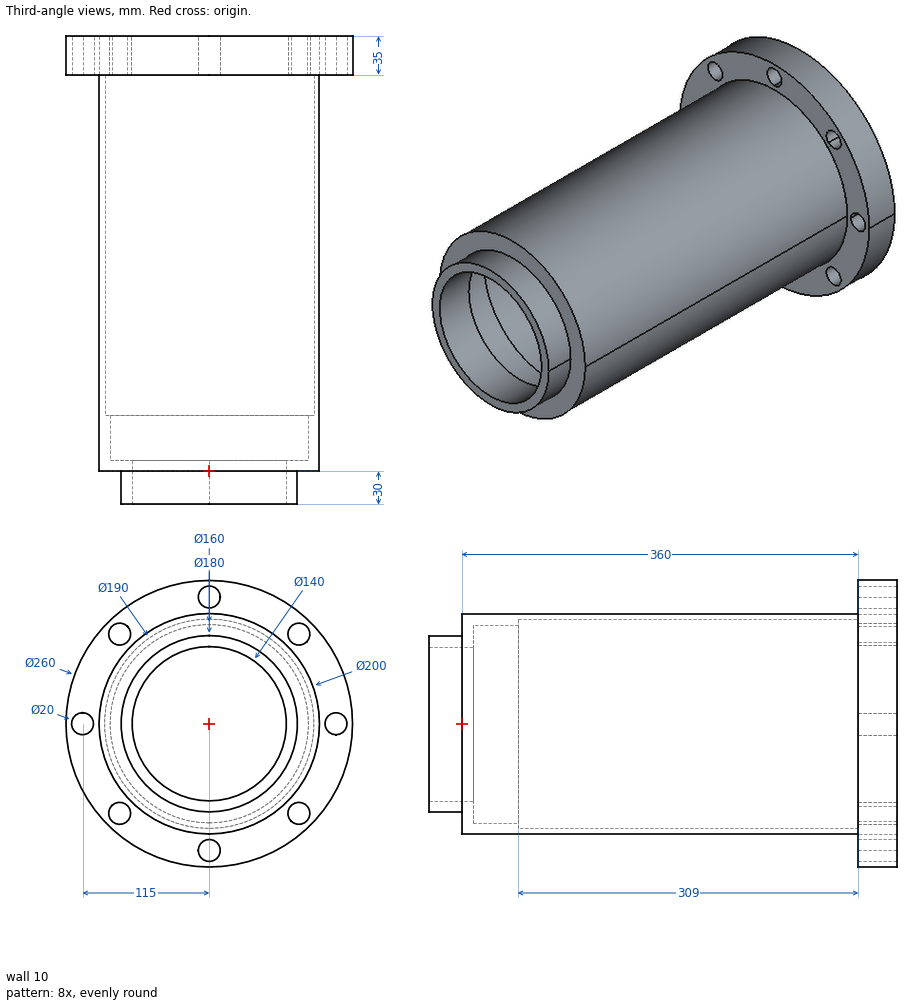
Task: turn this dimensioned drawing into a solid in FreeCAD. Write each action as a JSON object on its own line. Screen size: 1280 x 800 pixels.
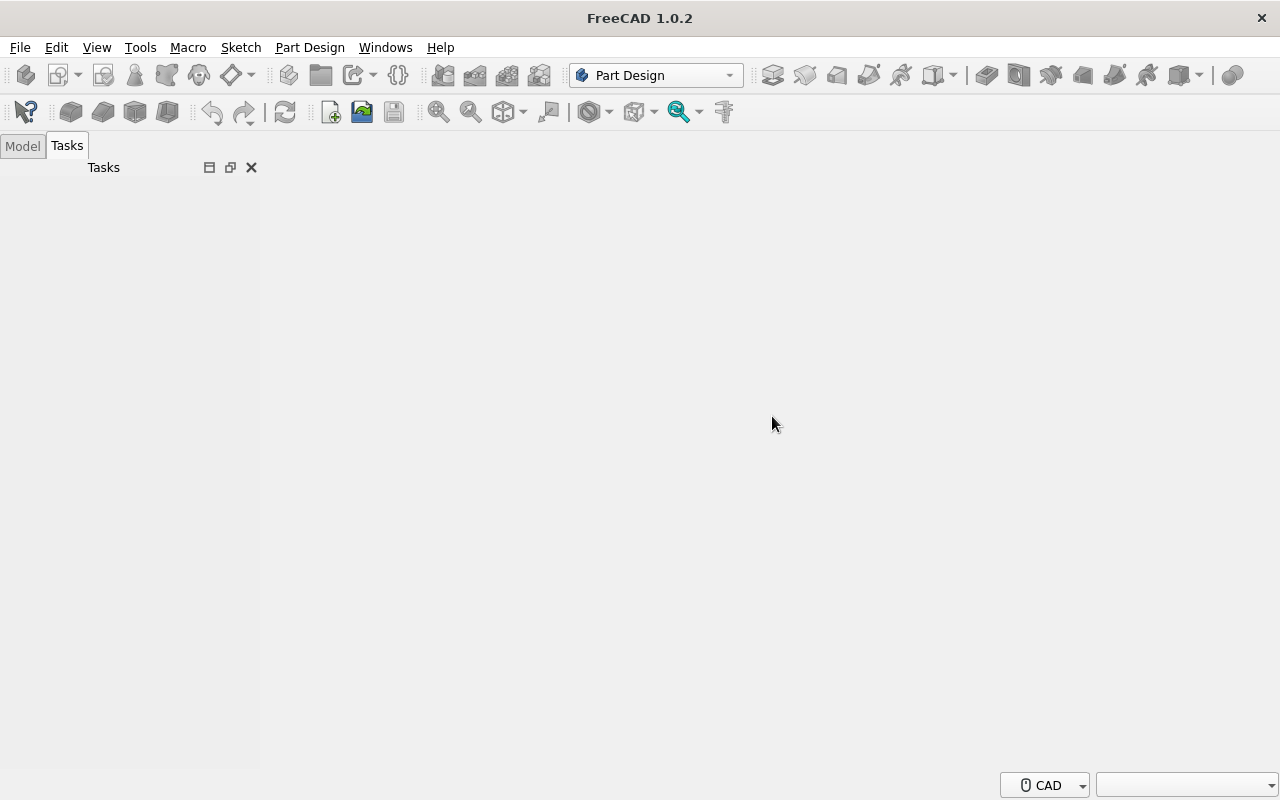
{"action": "key", "text": "ctrl+n"}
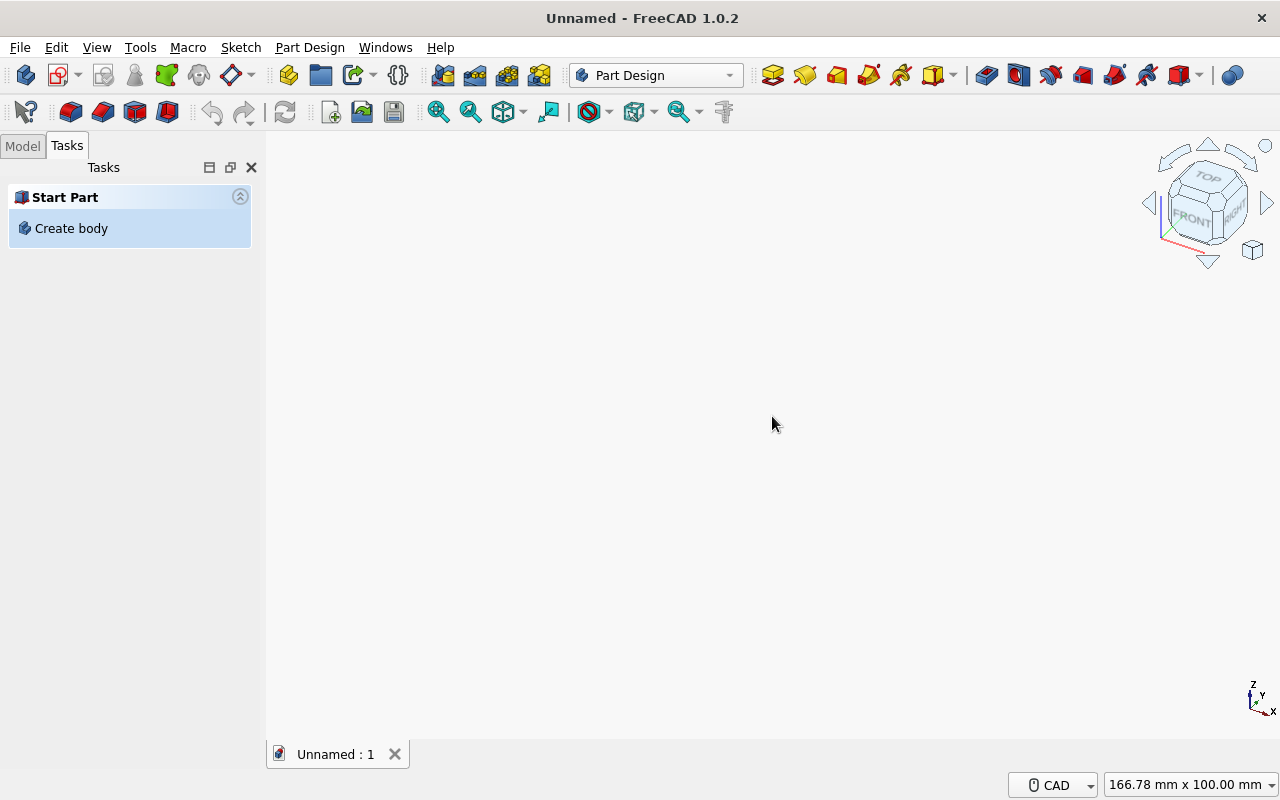
{"action": "left_click", "coordinate": [58, 76]}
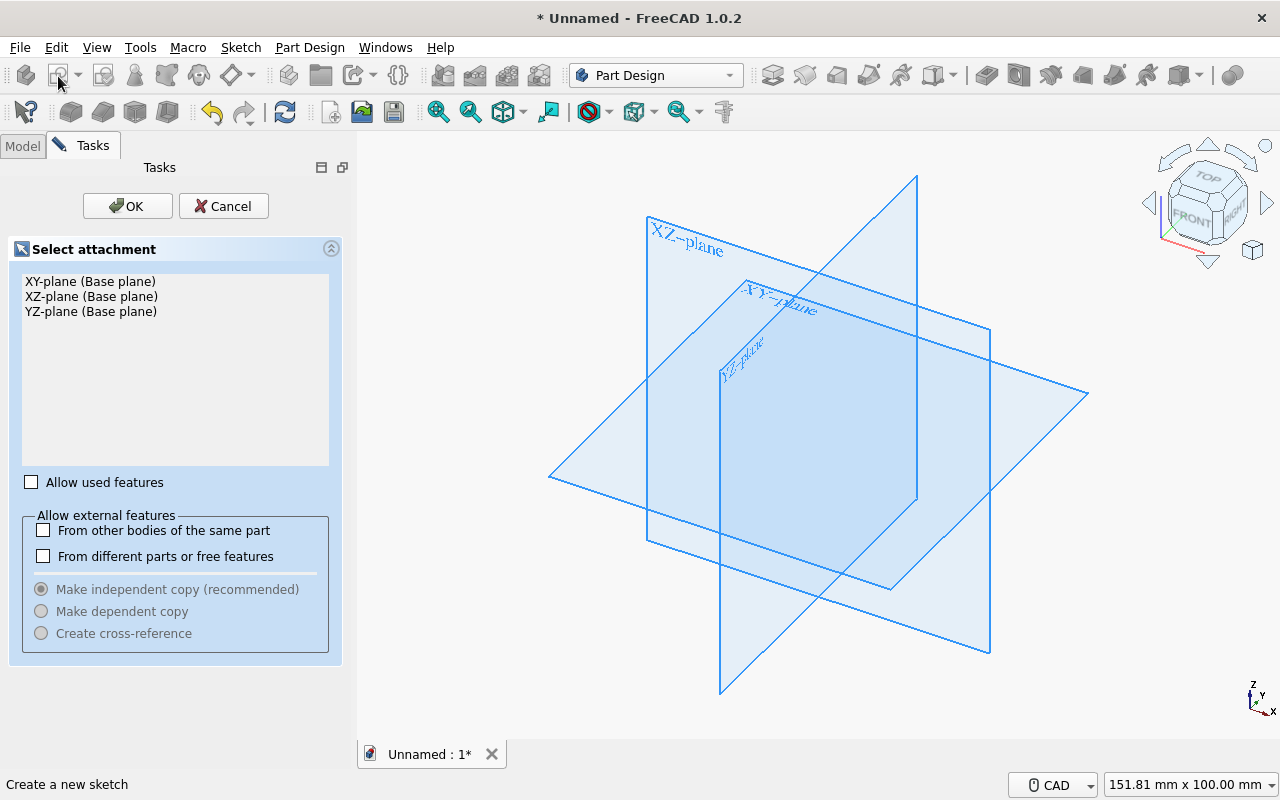
{"action": "left_click", "coordinate": [82, 296]}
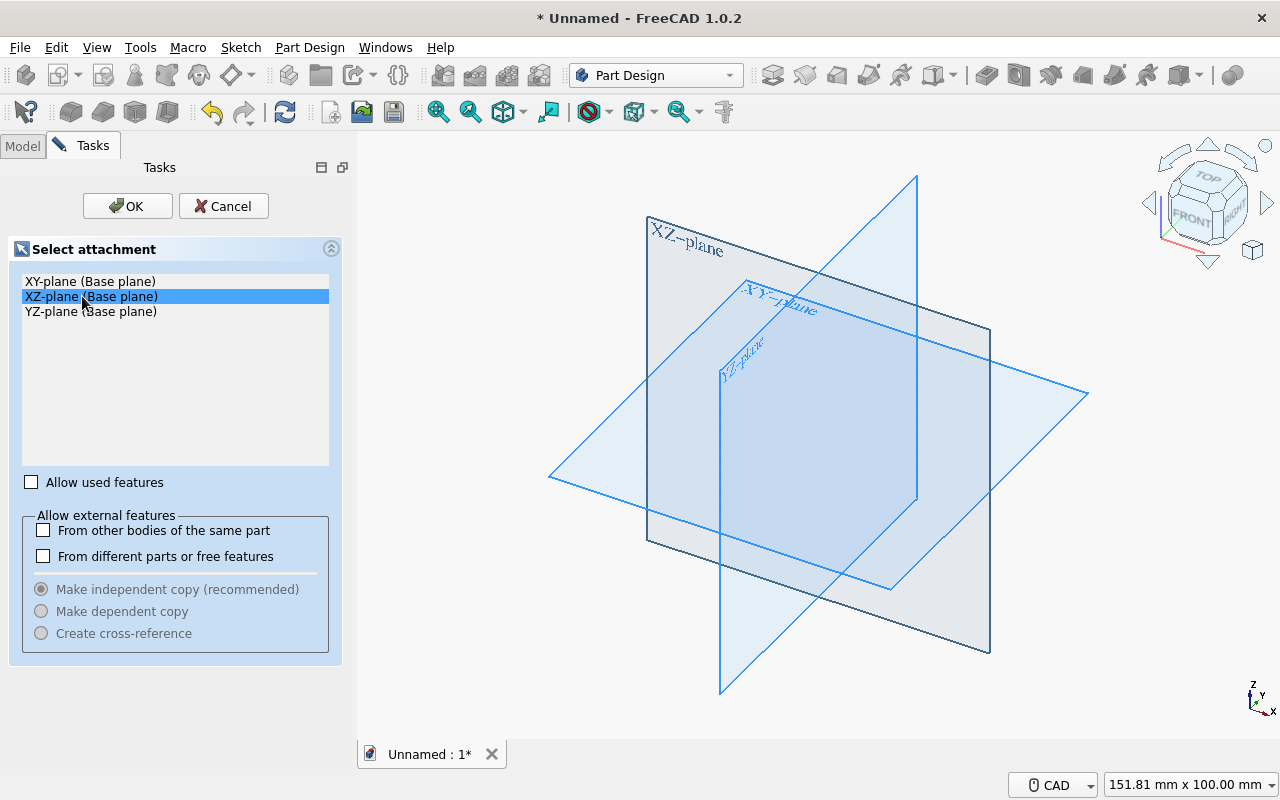
{"action": "left_click", "coordinate": [128, 206]}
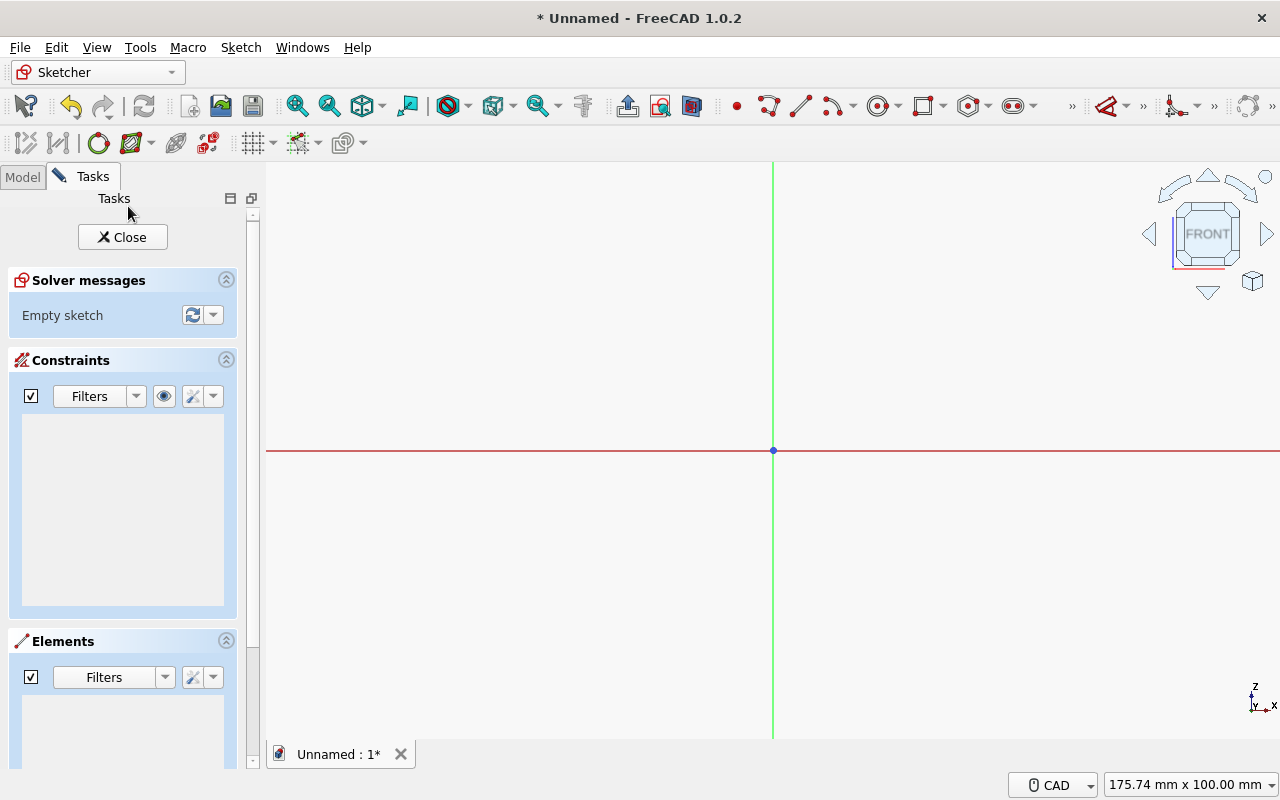
{"action": "scroll", "coordinate": [675, 450], "scroll_direction": "down", "scroll_amount": 6}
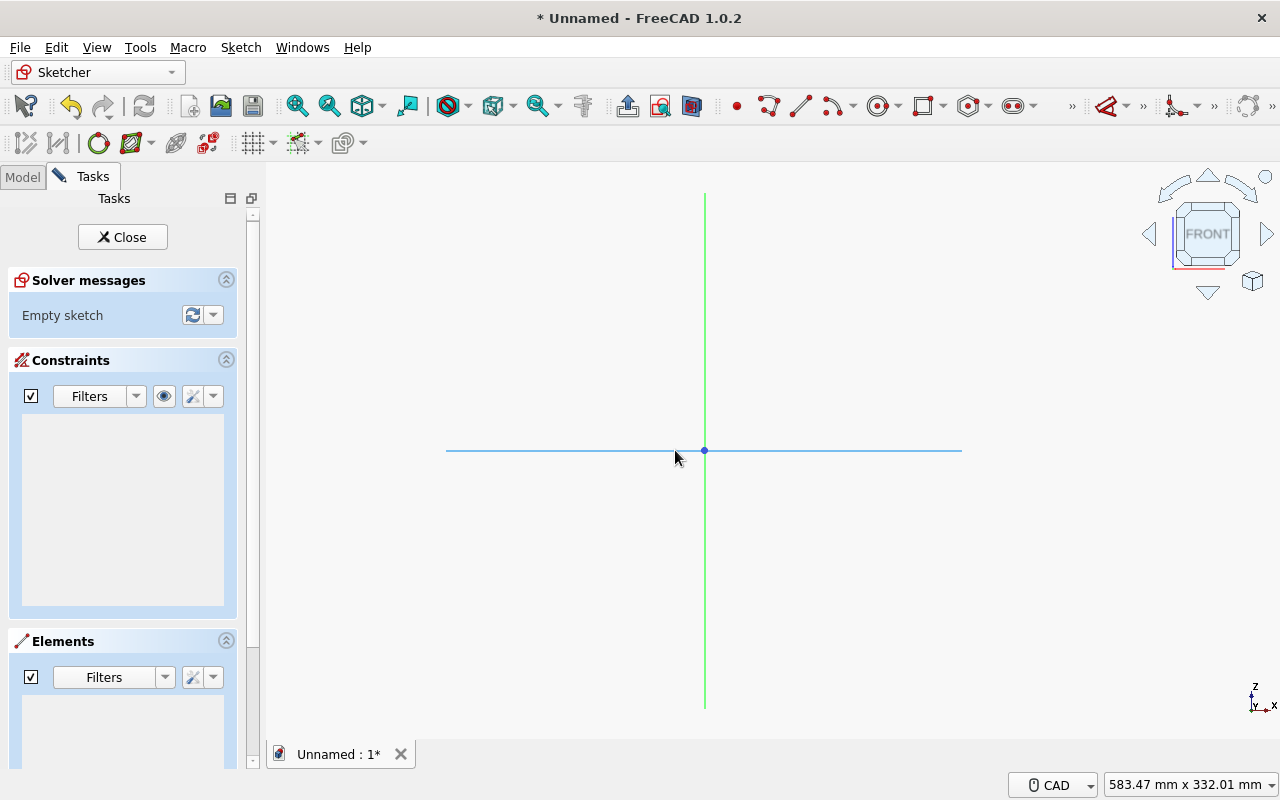
{"action": "left_click", "coordinate": [878, 106]}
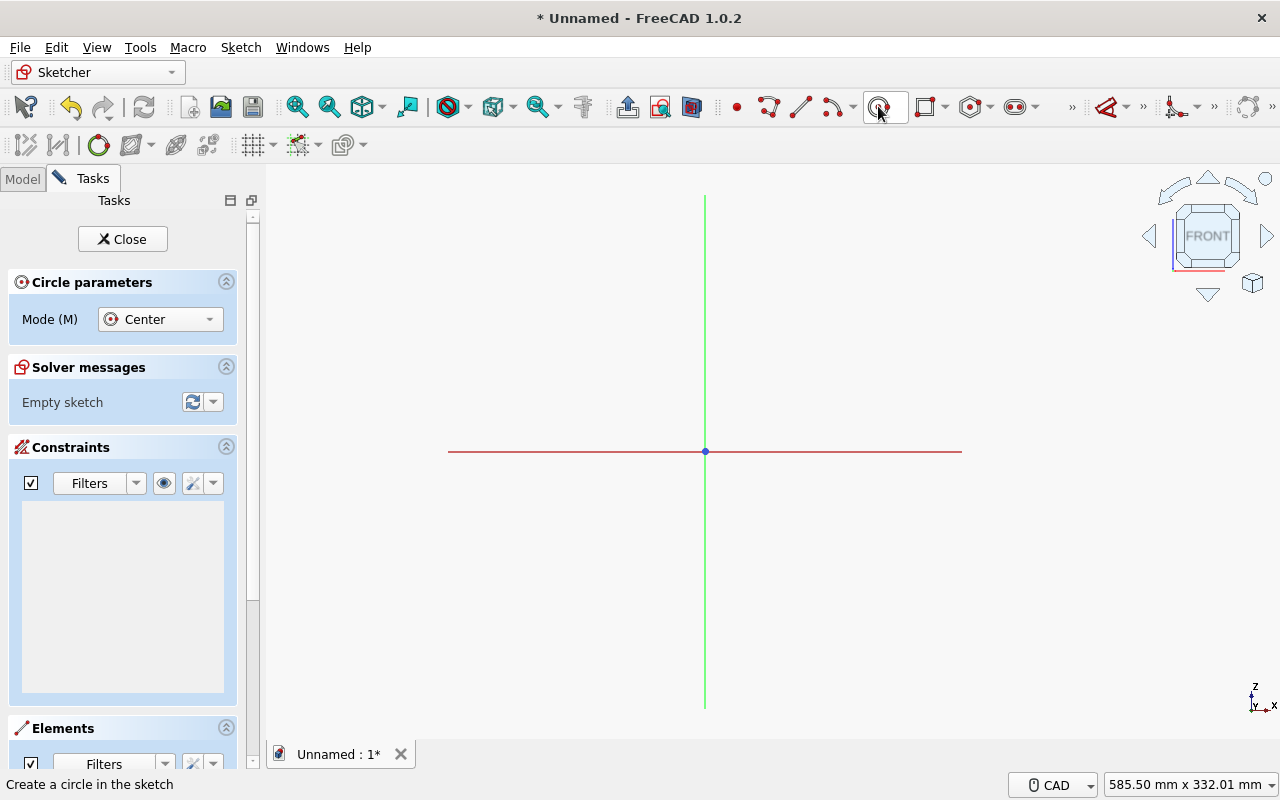
{"action": "left_click", "coordinate": [705, 452]}
{"action": "left_click", "coordinate": [827, 329]}
{"action": "key", "text": "Escape"}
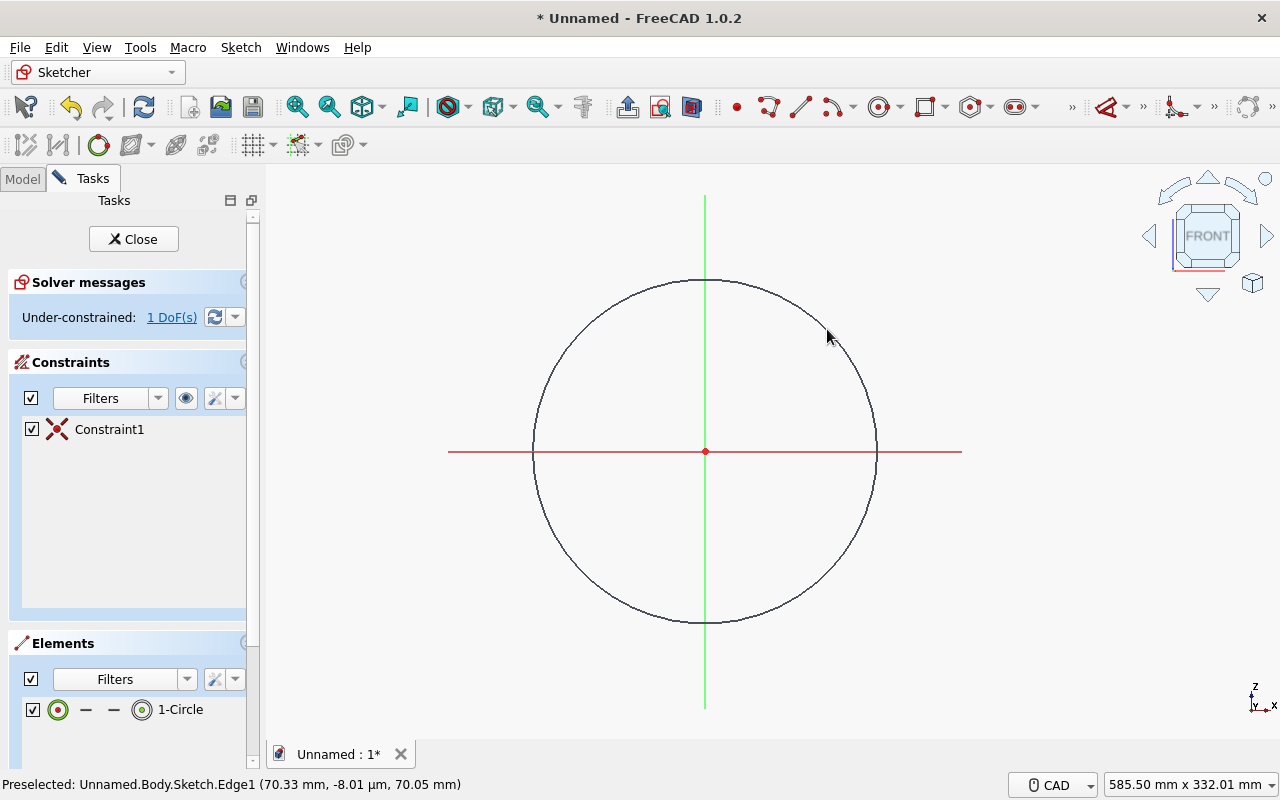
{"action": "key", "text": "d"}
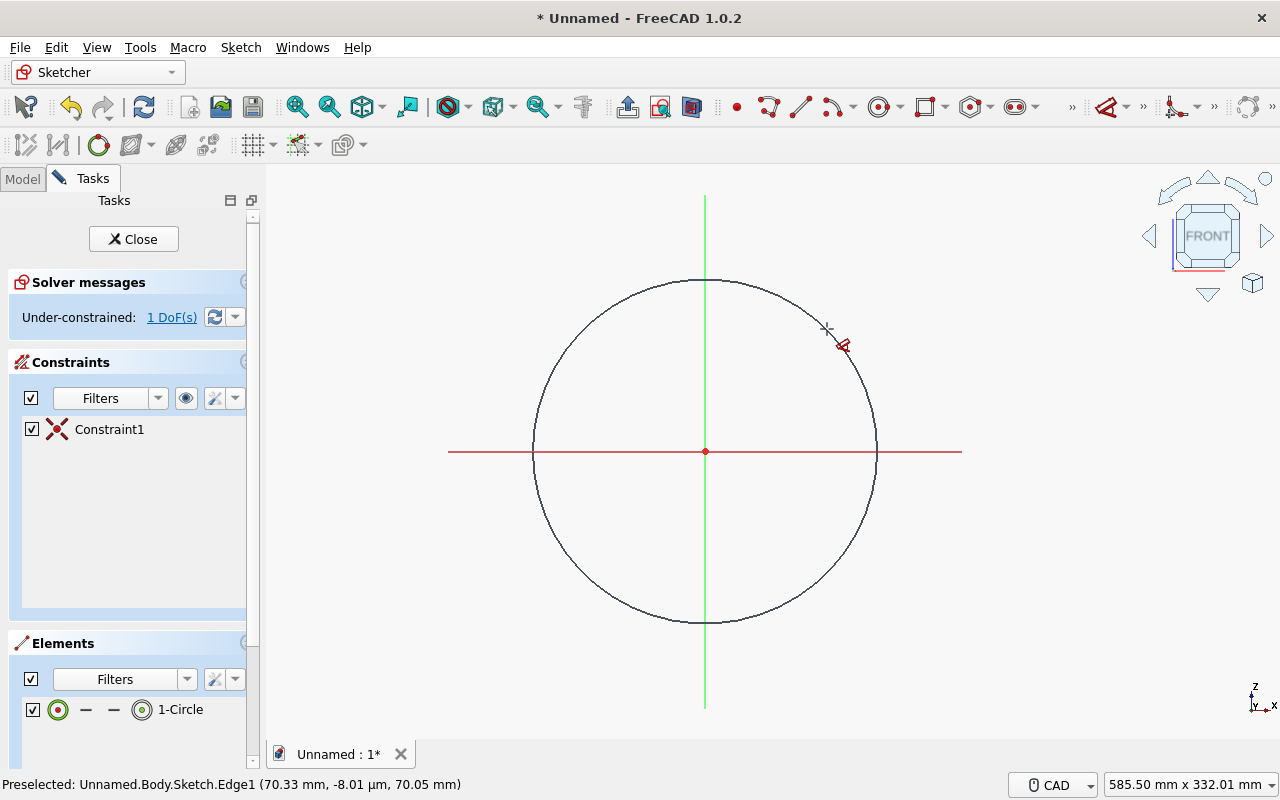
{"action": "left_click", "coordinate": [826, 329]}
{"action": "left_click", "coordinate": [848, 306]}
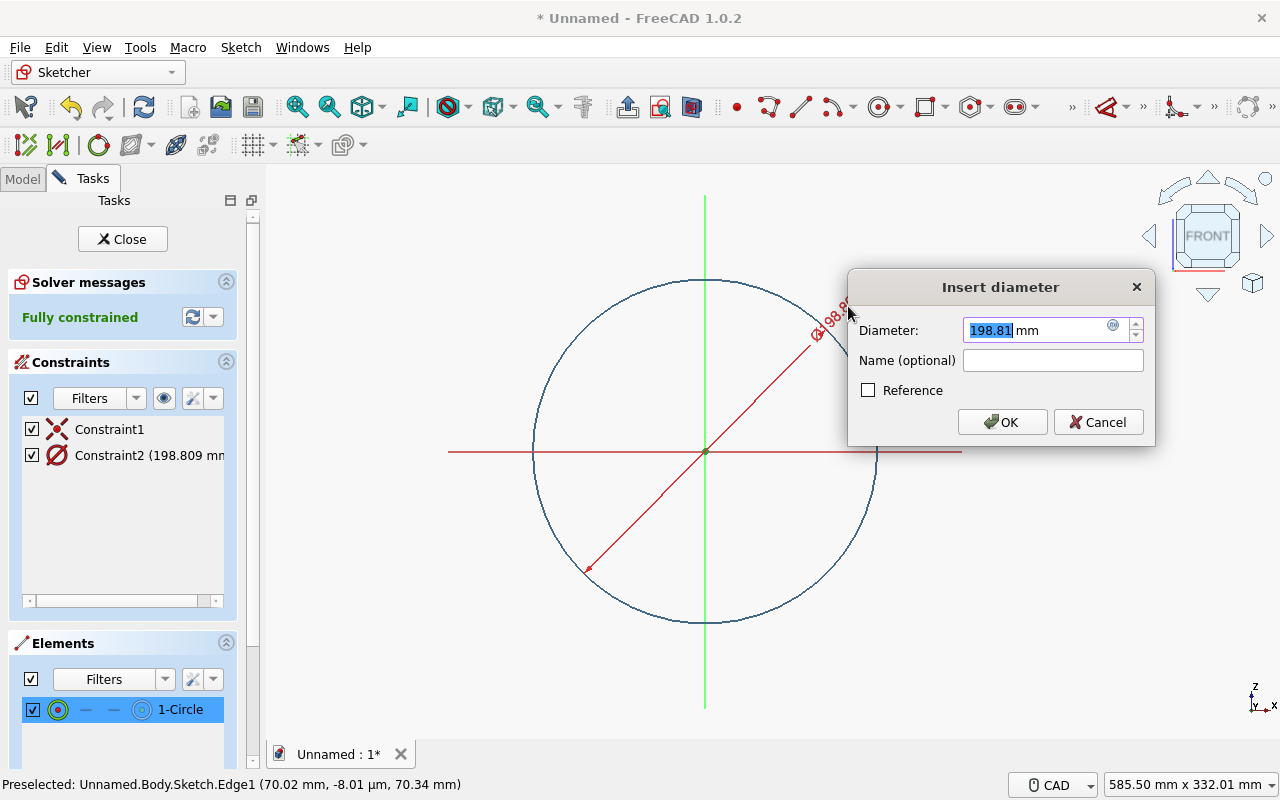
{"action": "type", "text": "200"}
{"action": "key", "text": "Return"}
{"action": "key", "text": "Escape"}